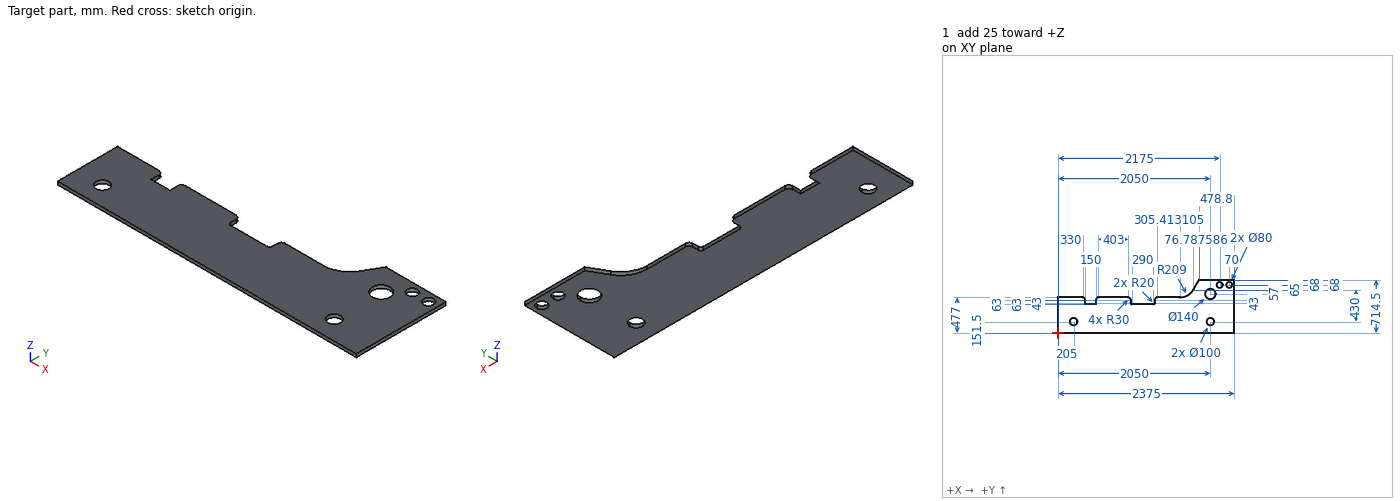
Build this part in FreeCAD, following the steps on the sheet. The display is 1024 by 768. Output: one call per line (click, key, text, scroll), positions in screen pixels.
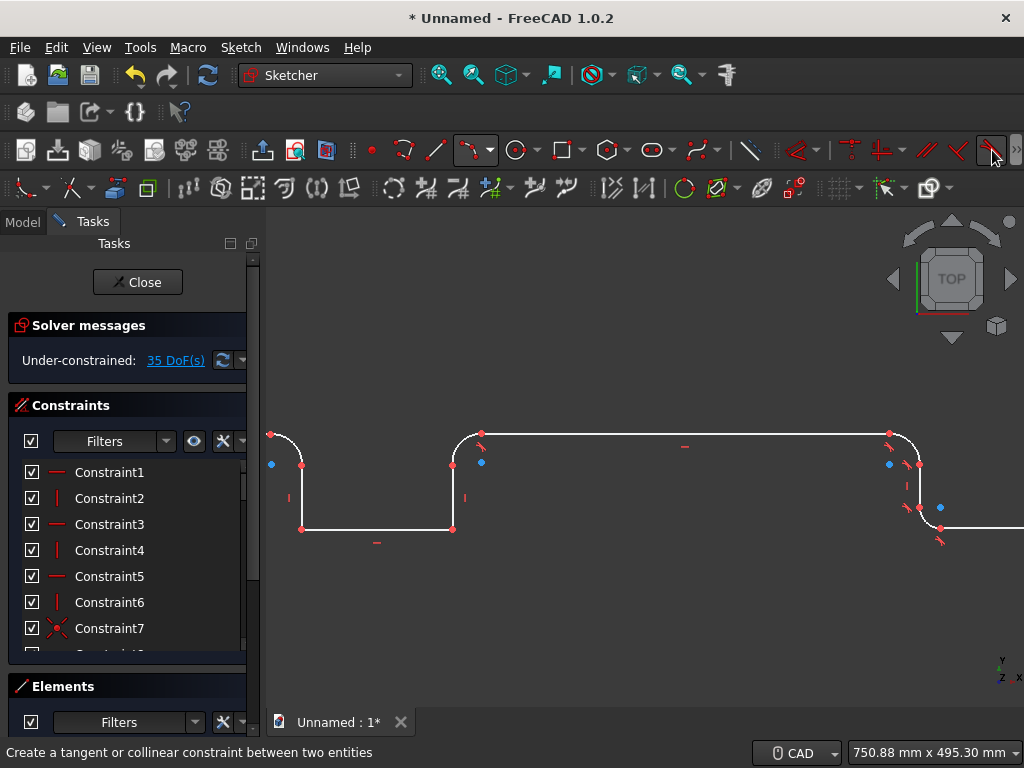
click(453, 485)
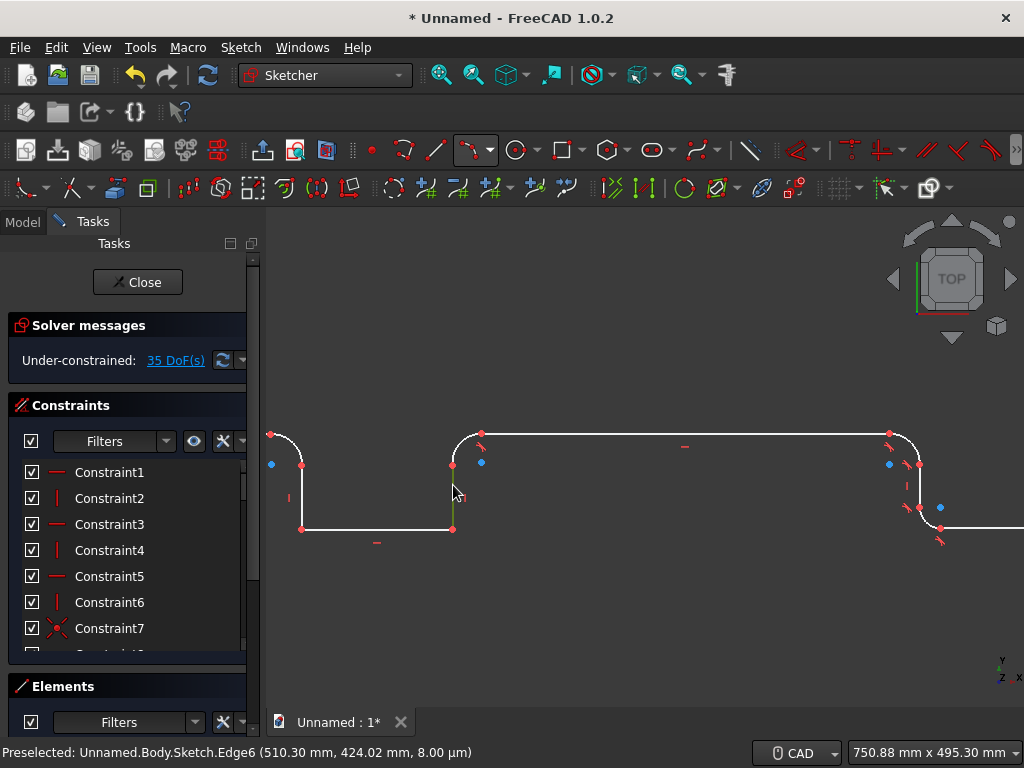
click(468, 437)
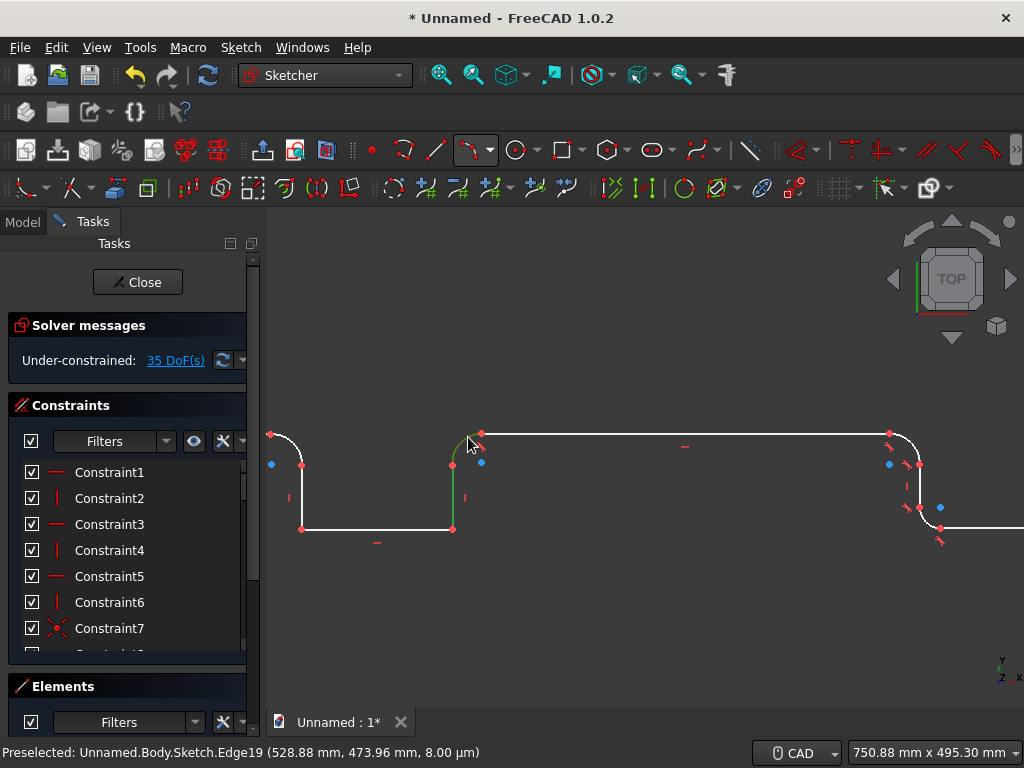
click(992, 150)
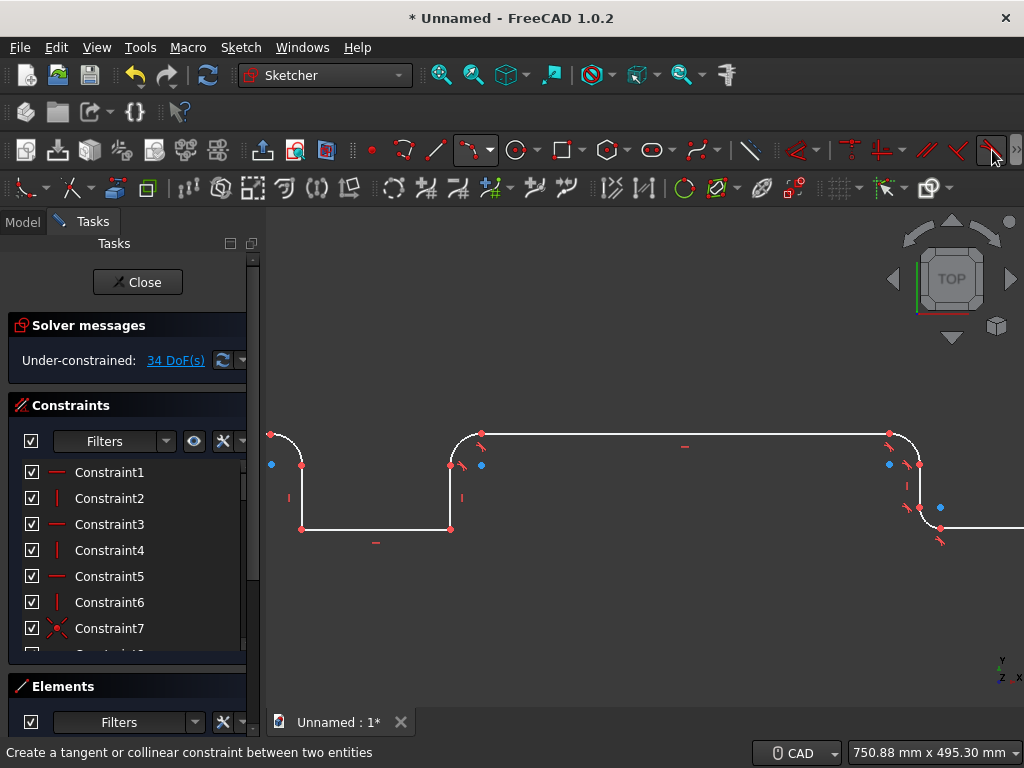
click(302, 510)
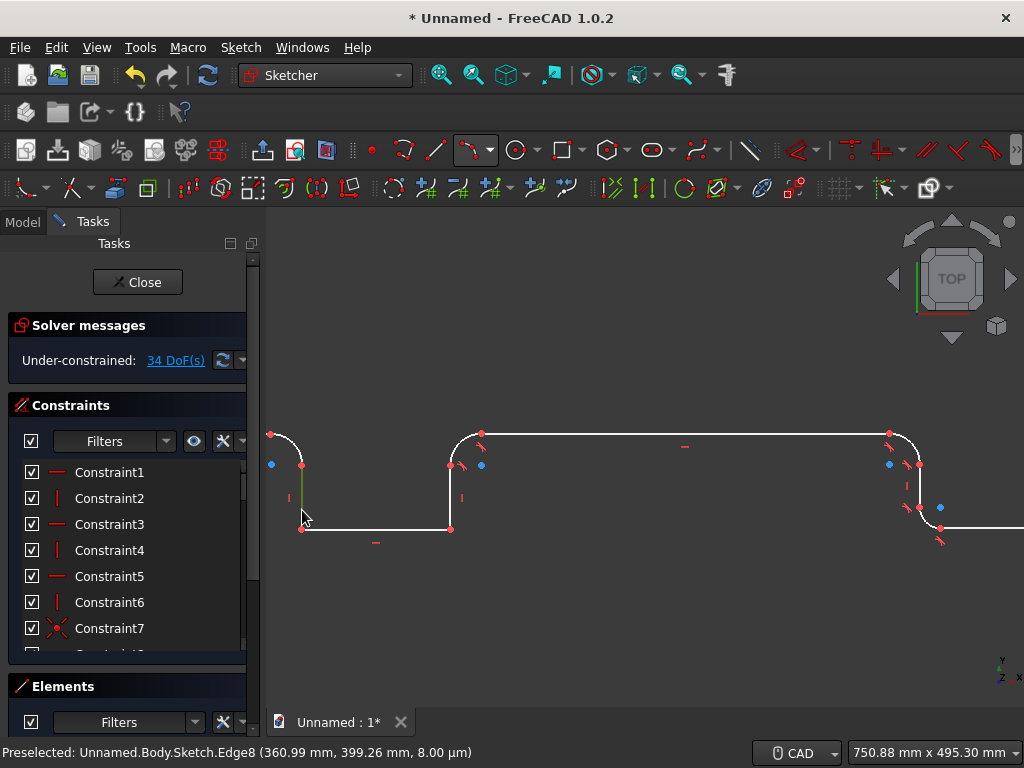
click(299, 451)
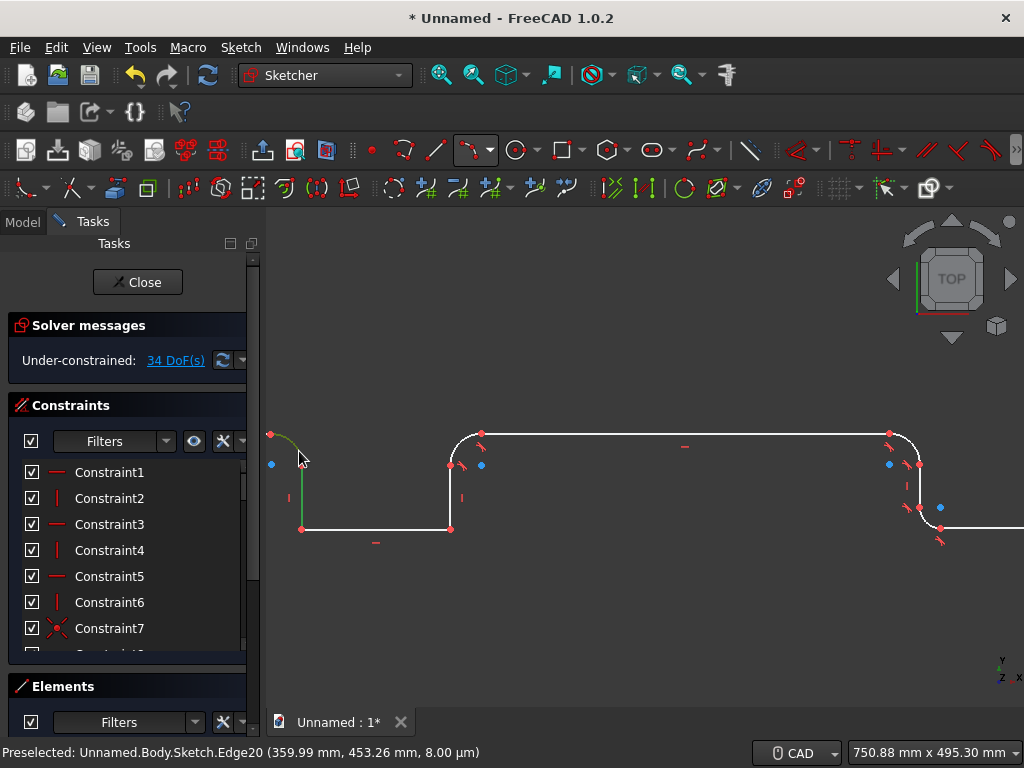
click(992, 150)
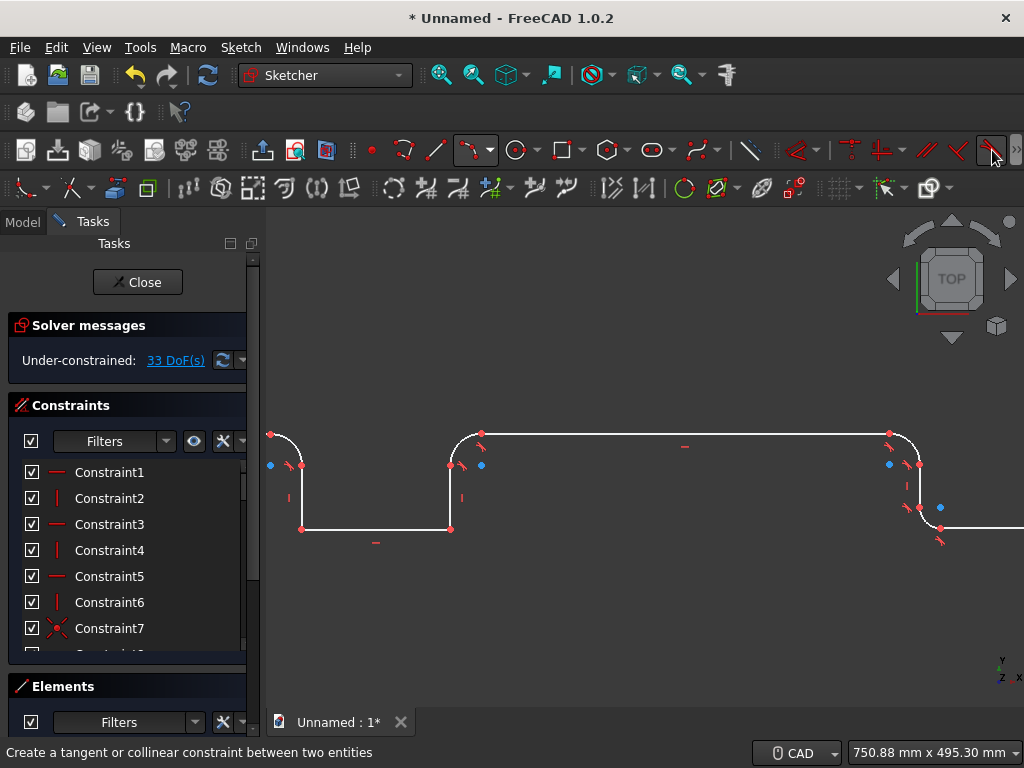
scroll(466, 438, down, 9)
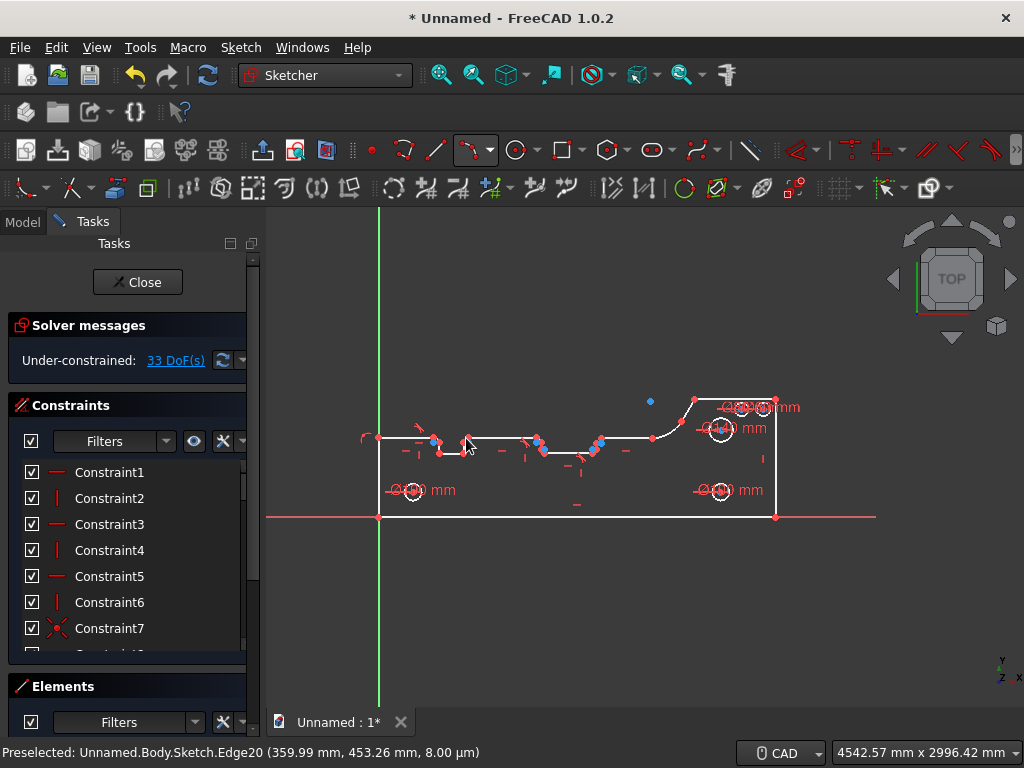
click(395, 438)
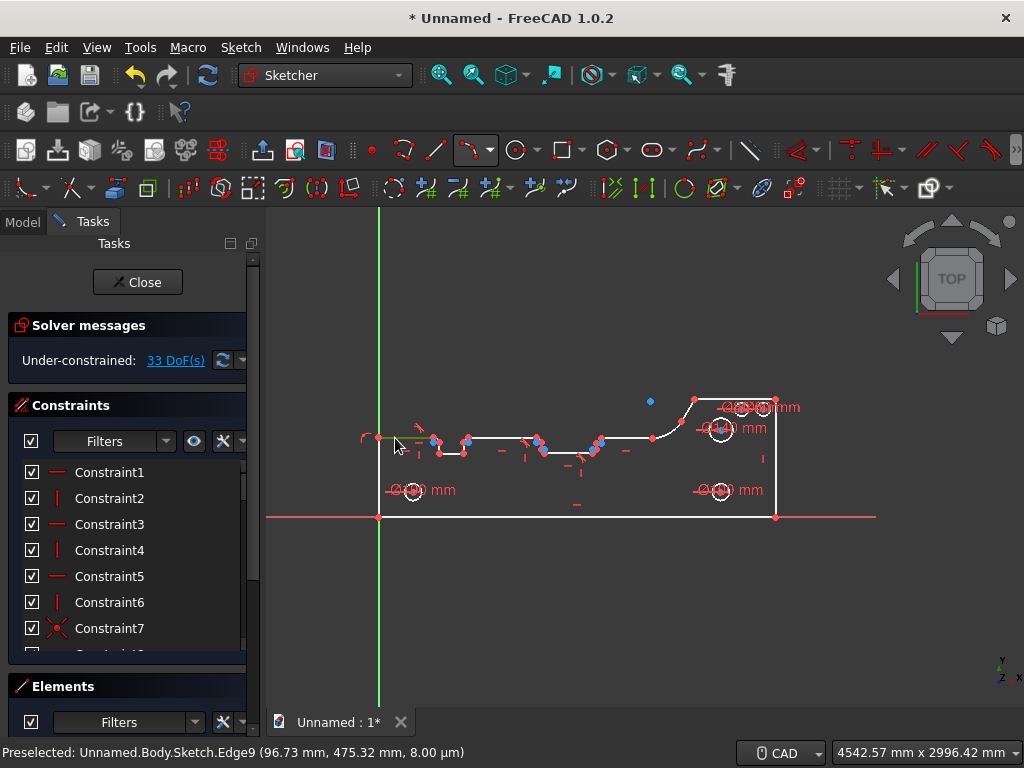
scroll(438, 439, up, 7)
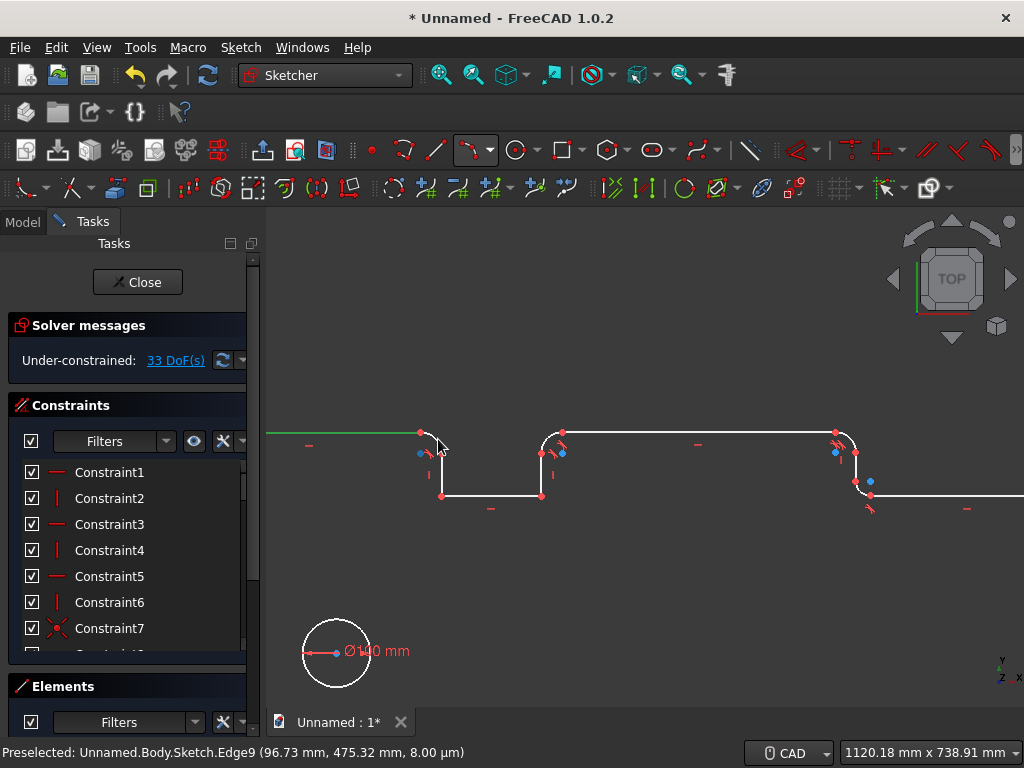
click(436, 439)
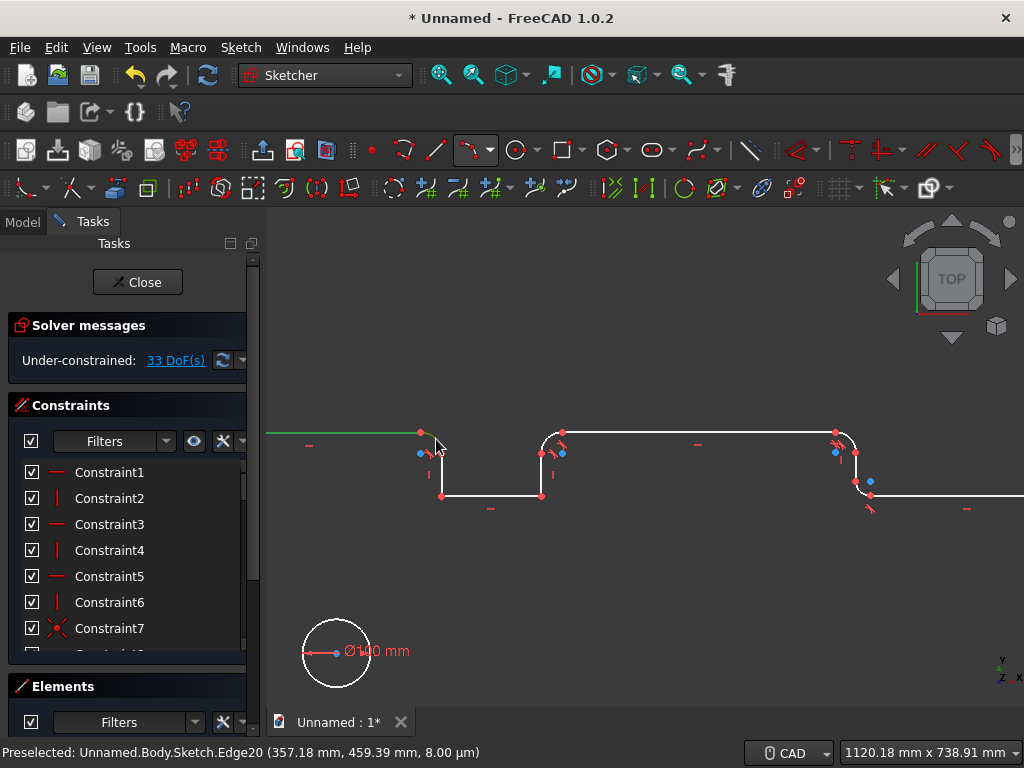
click(992, 150)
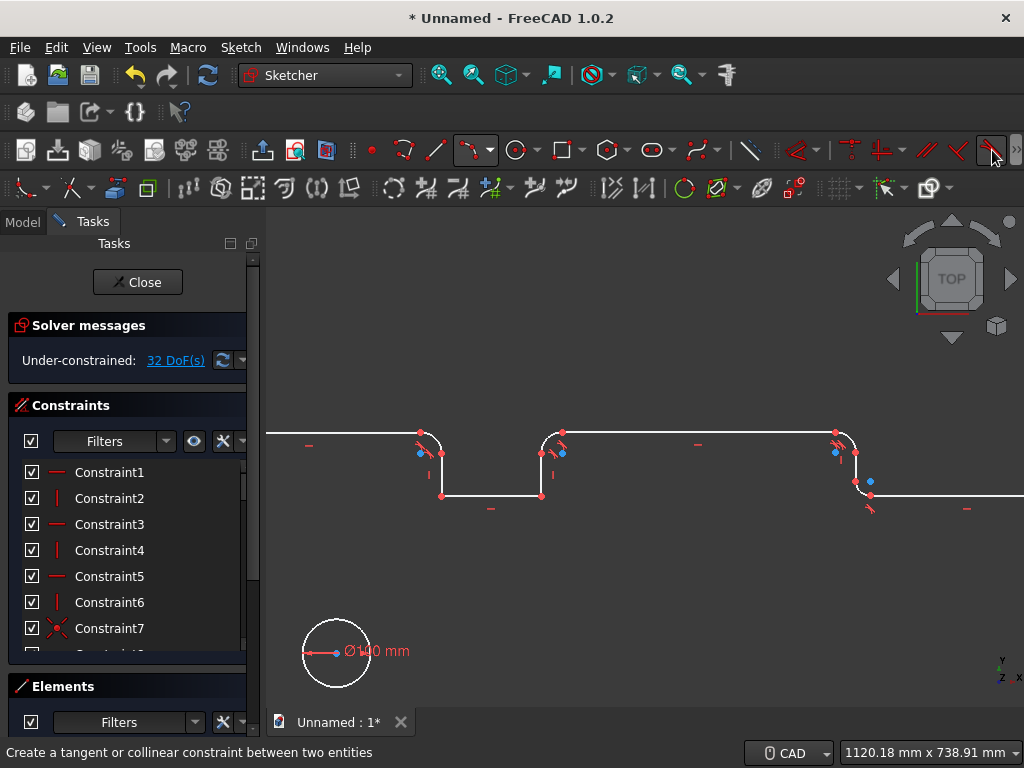
scroll(438, 439, down, 7)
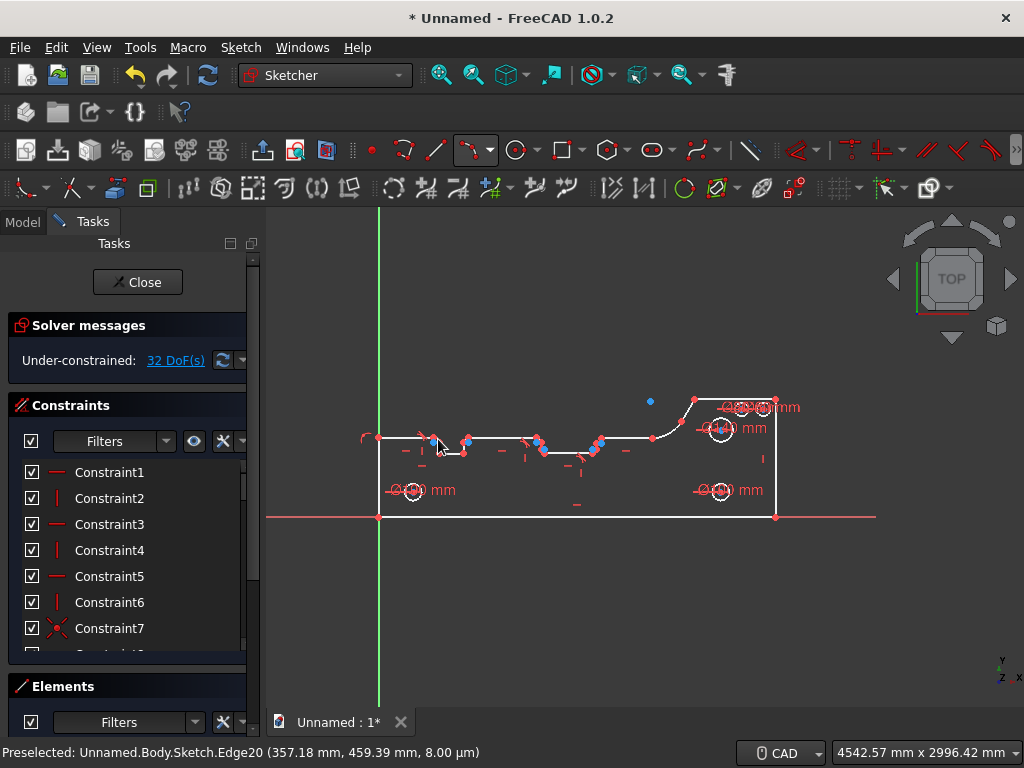
scroll(595, 452, up, 9)